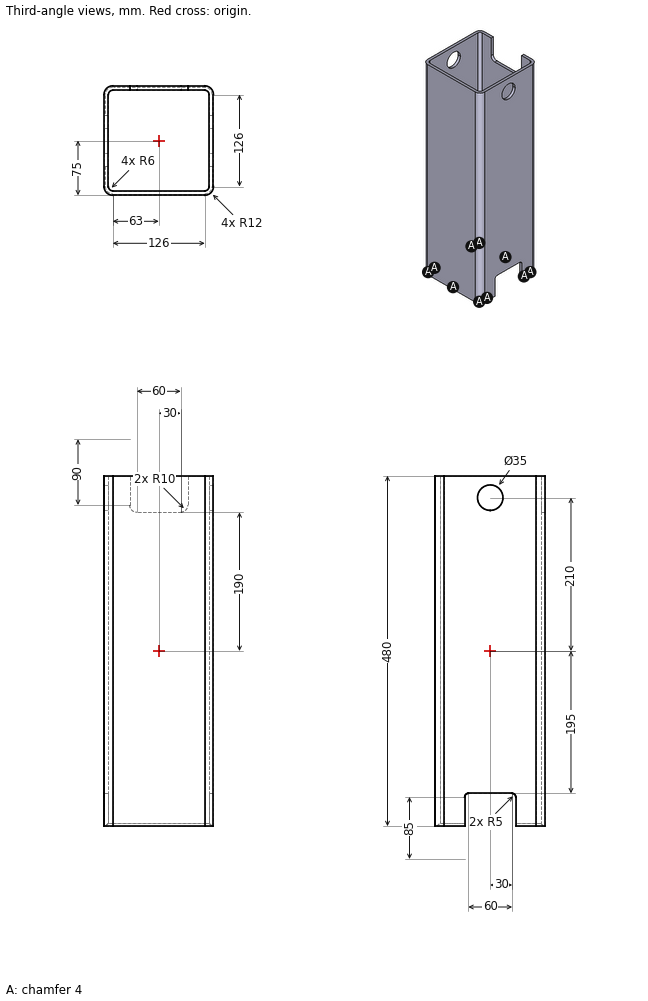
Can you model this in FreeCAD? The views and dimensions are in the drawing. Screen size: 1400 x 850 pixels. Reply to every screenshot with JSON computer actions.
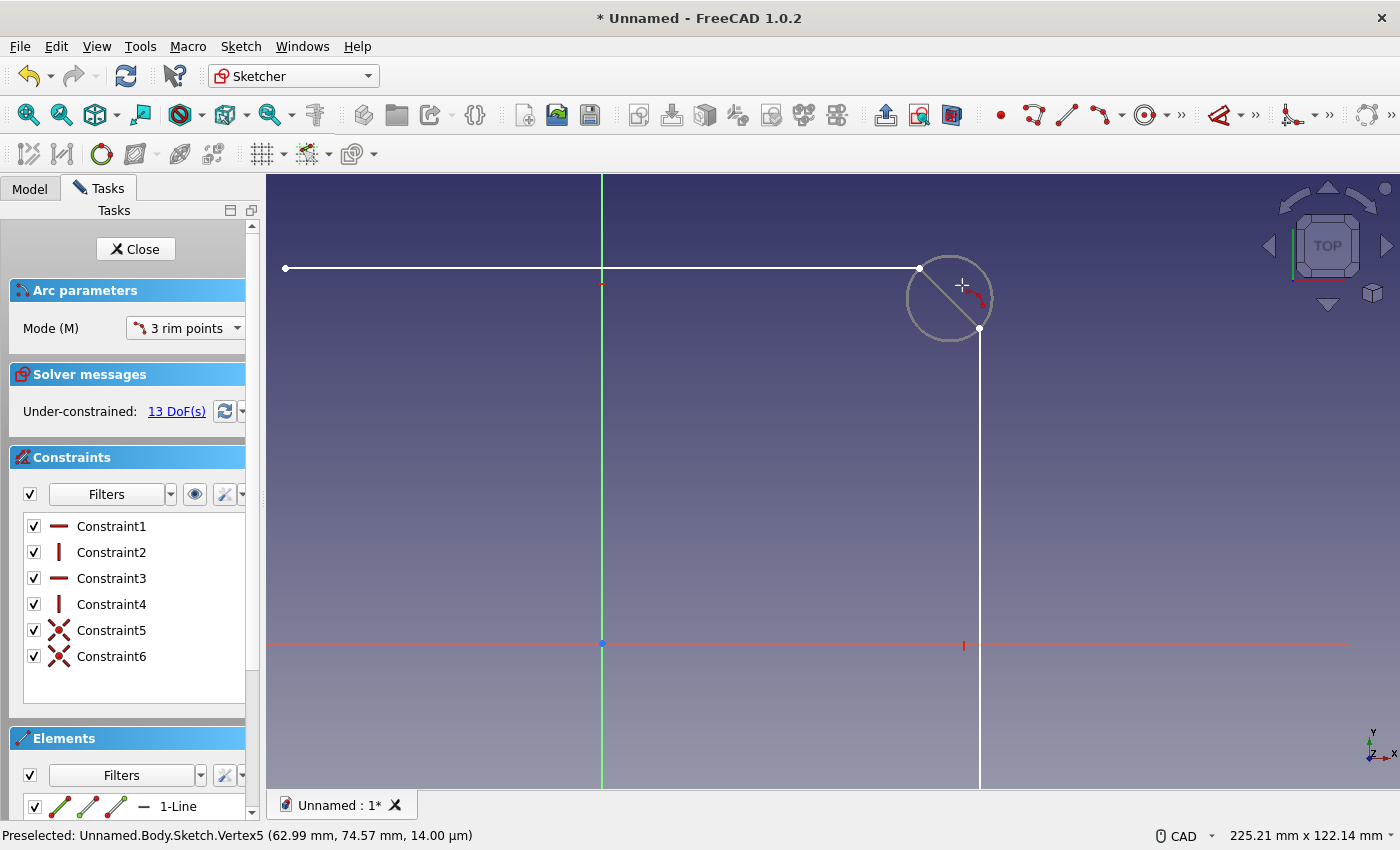
{"action": "left_click", "coordinate": [962, 284]}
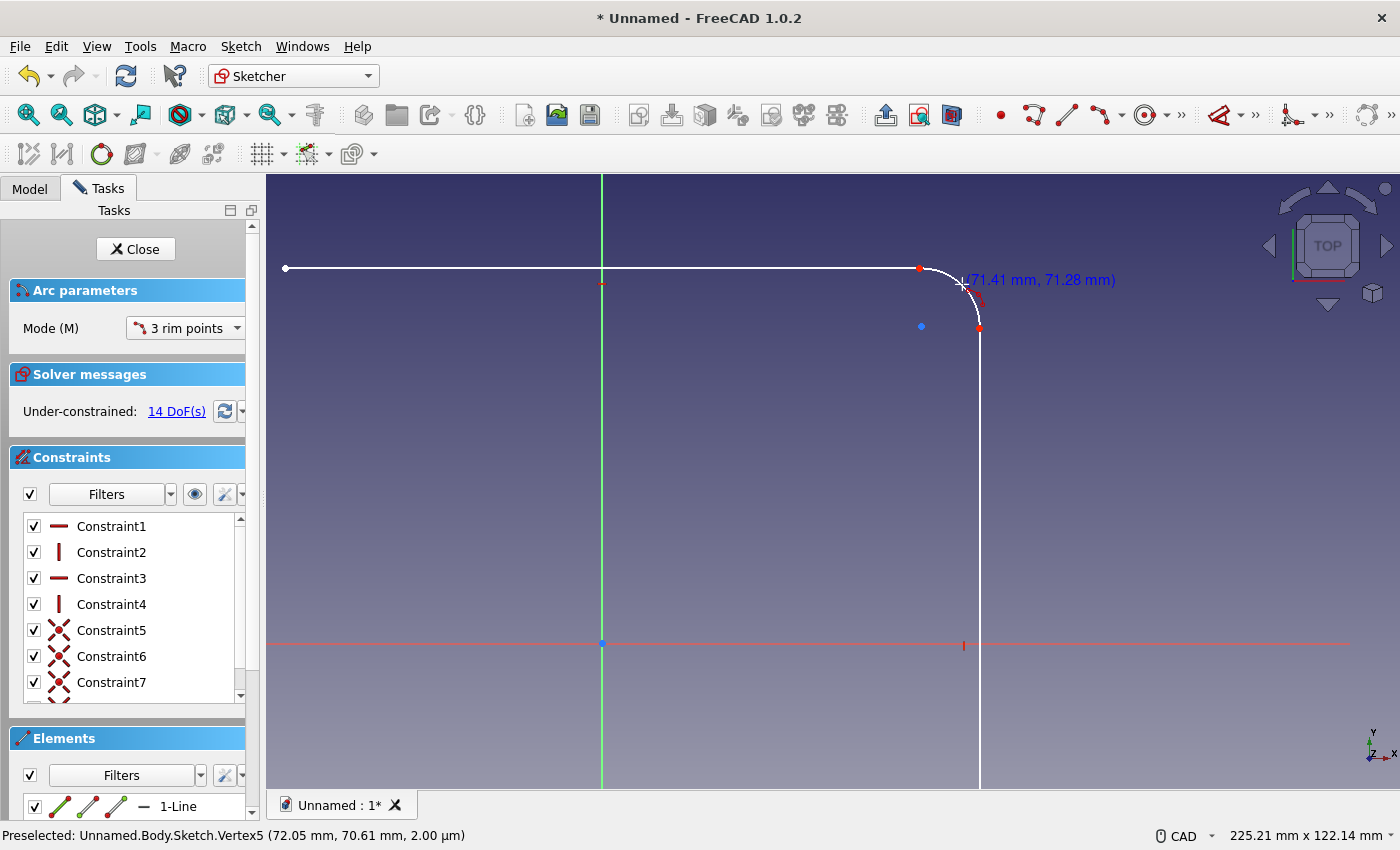
{"action": "scroll", "coordinate": [962, 284], "scroll_direction": "down", "scroll_amount": 3}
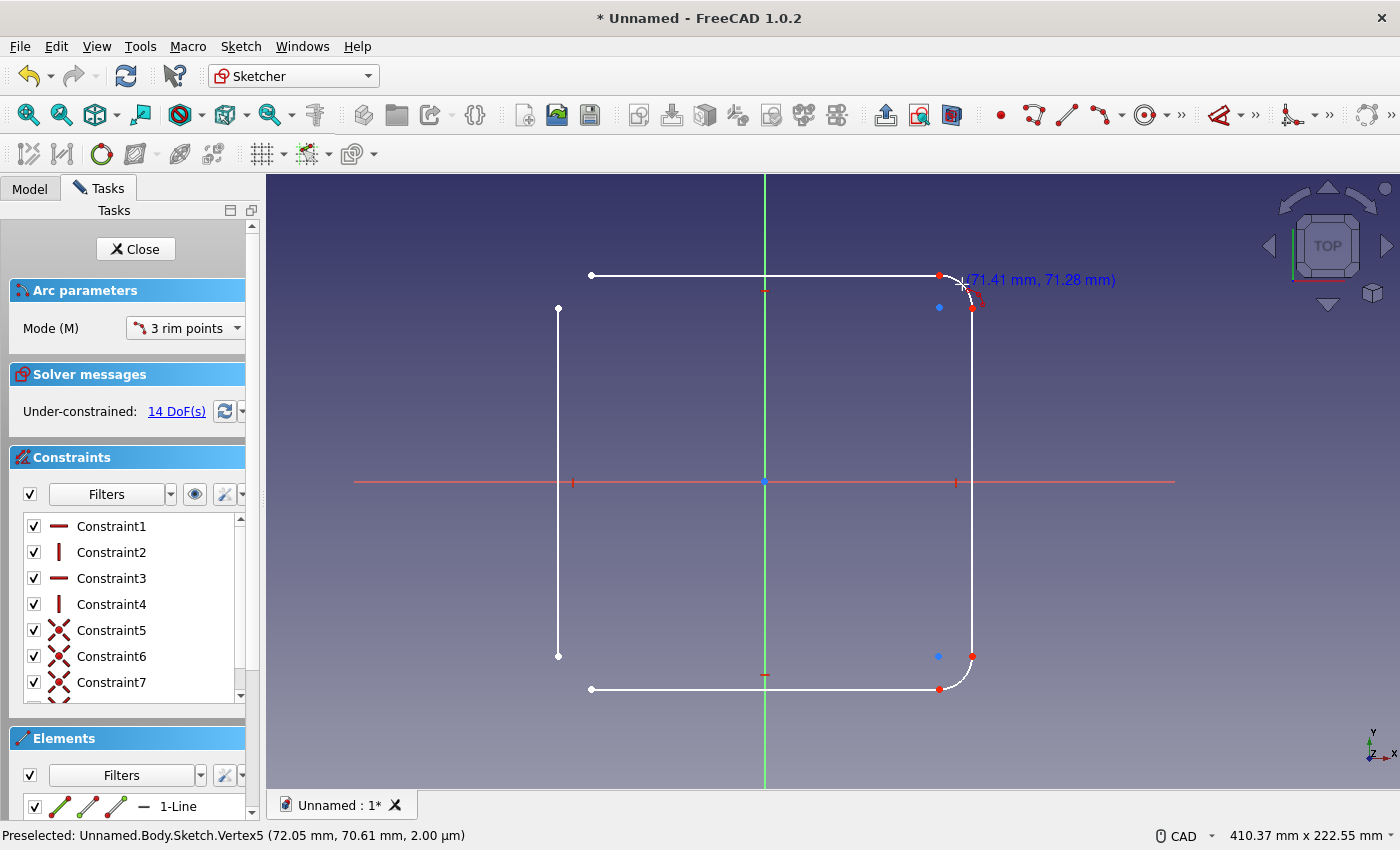
{"action": "left_click", "coordinate": [591, 276]}
{"action": "left_click", "coordinate": [558, 309]}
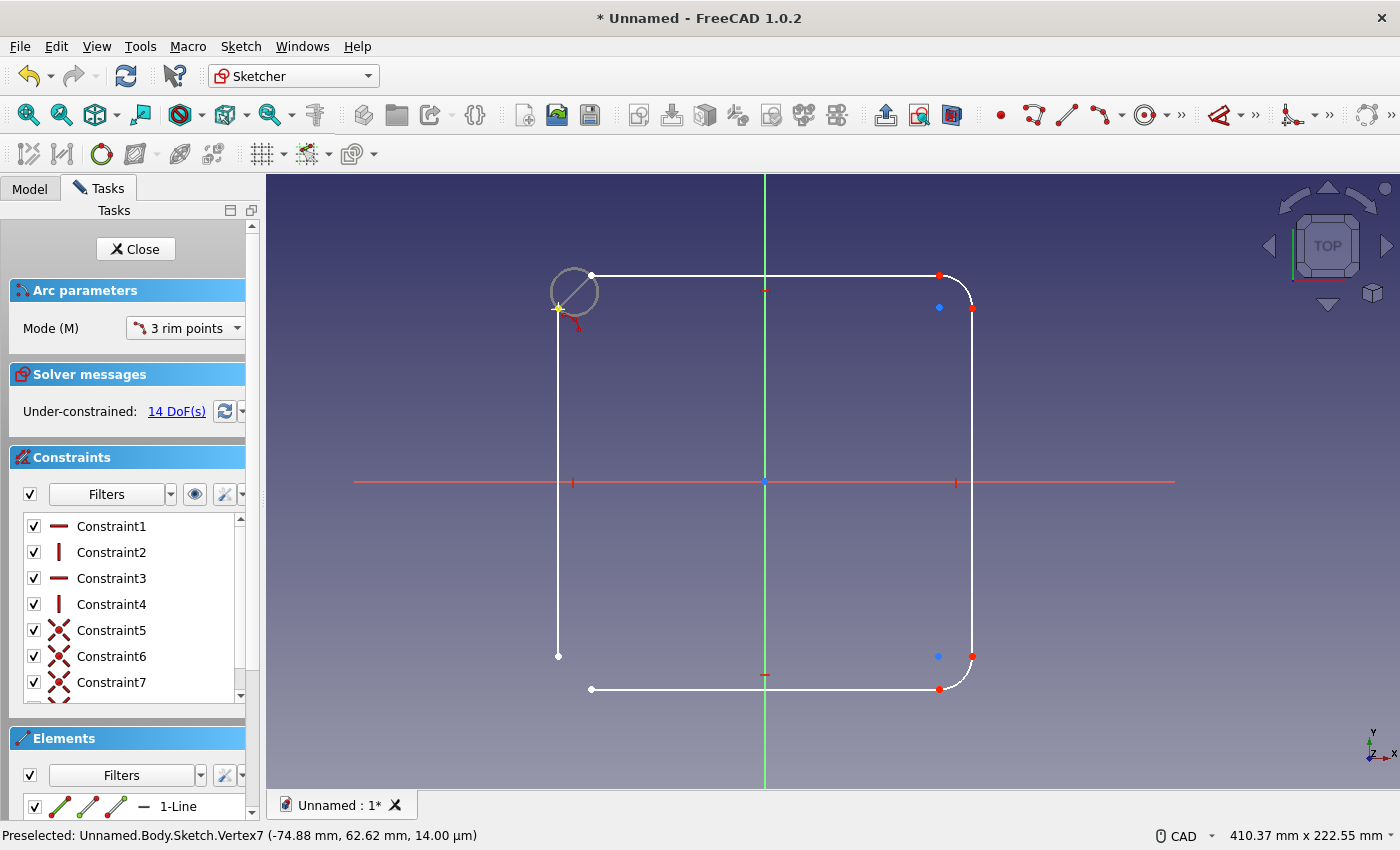
{"action": "scroll", "coordinate": [567, 284], "scroll_direction": "up", "scroll_amount": 3}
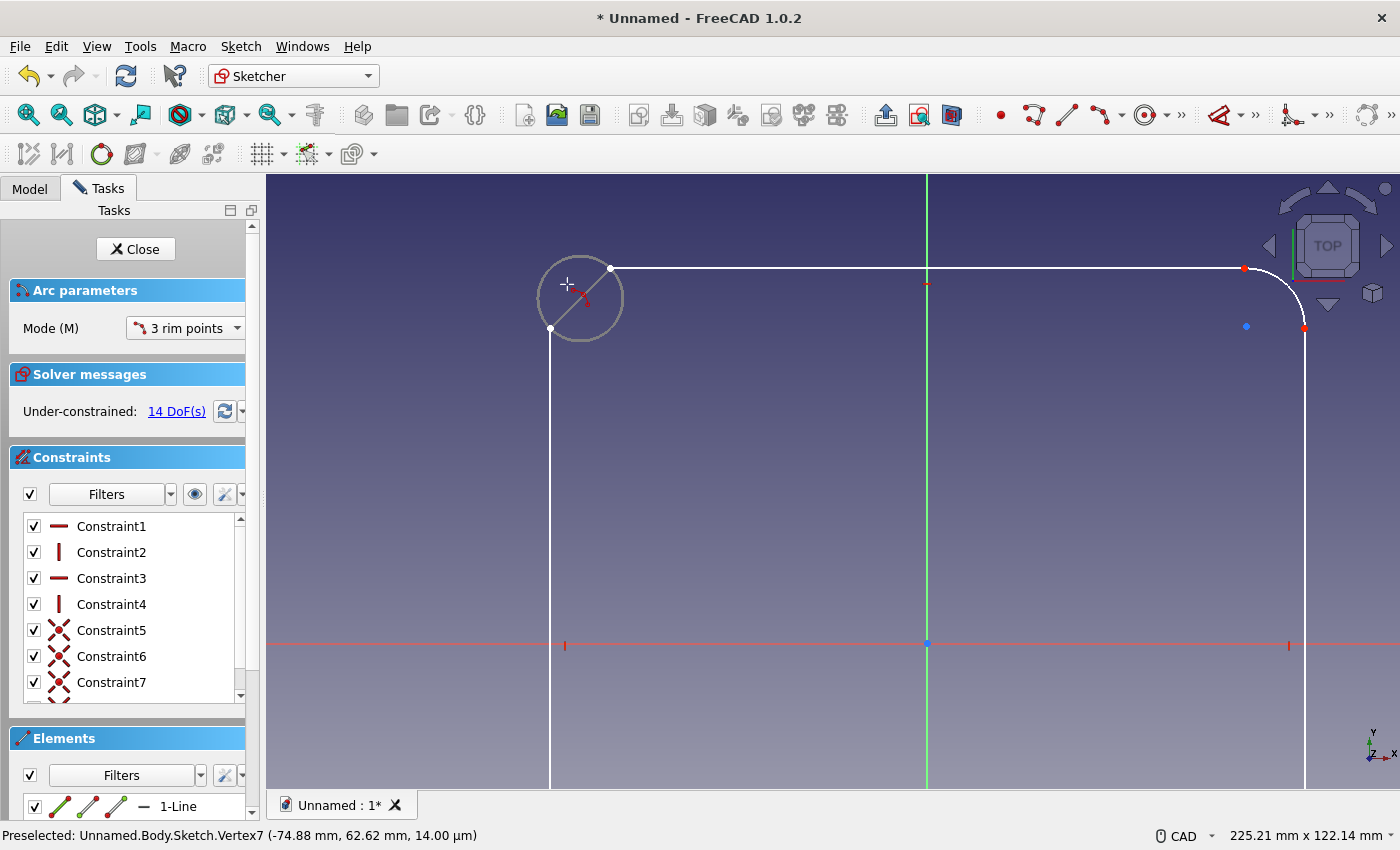
{"action": "left_click", "coordinate": [567, 284]}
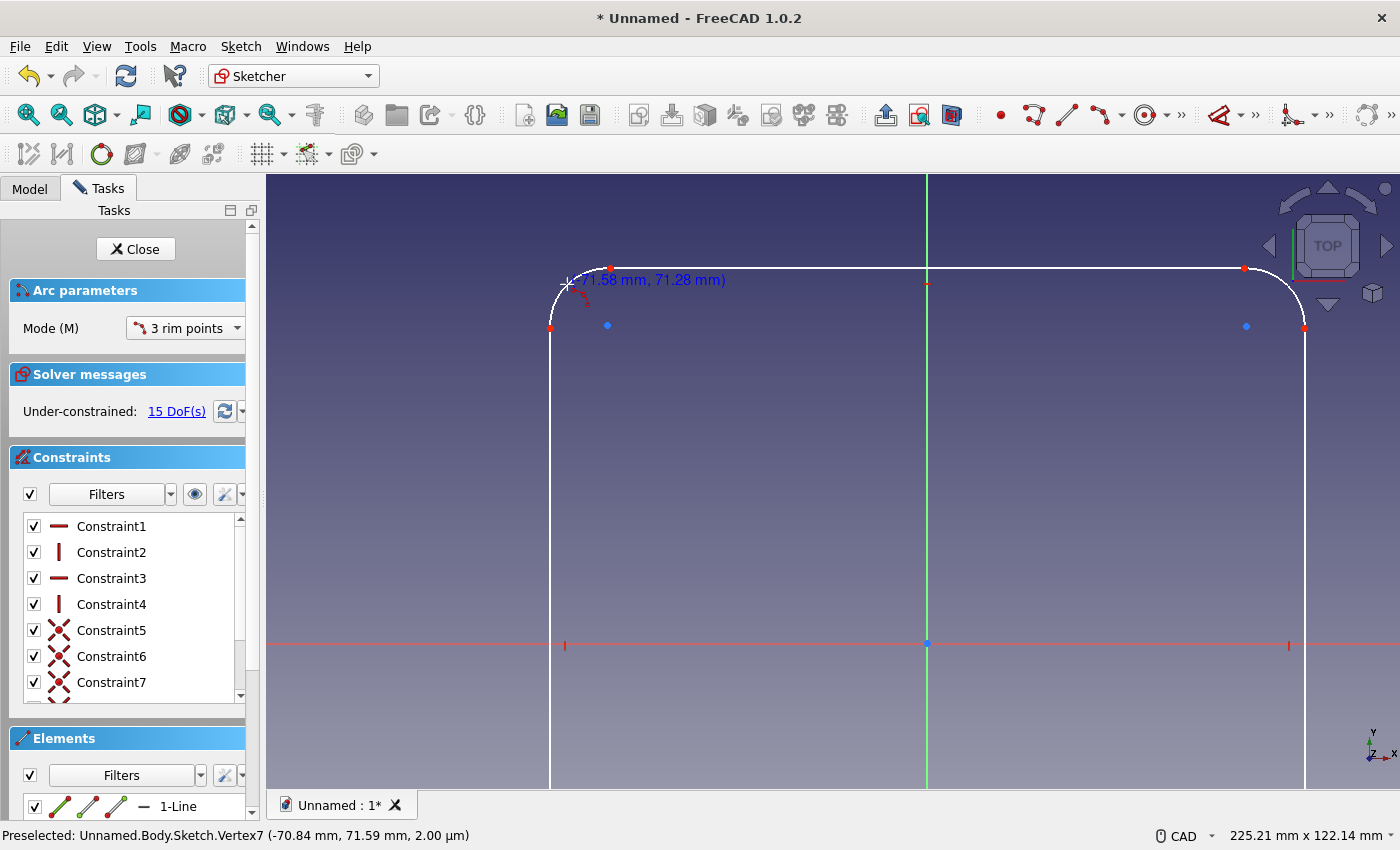
{"action": "scroll", "coordinate": [566, 284], "scroll_direction": "down", "scroll_amount": 3}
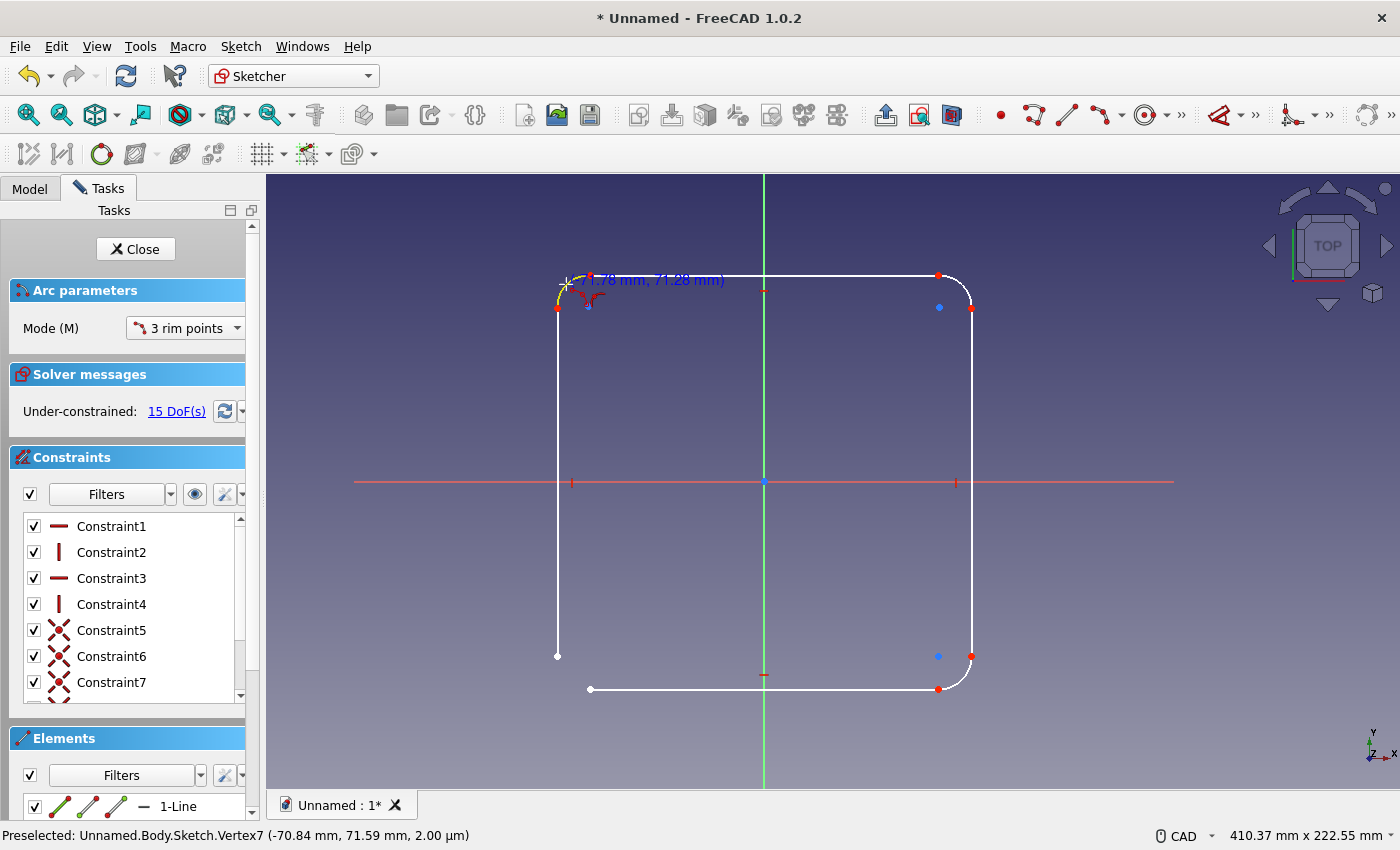
{"action": "left_click", "coordinate": [558, 657]}
{"action": "left_click", "coordinate": [591, 690]}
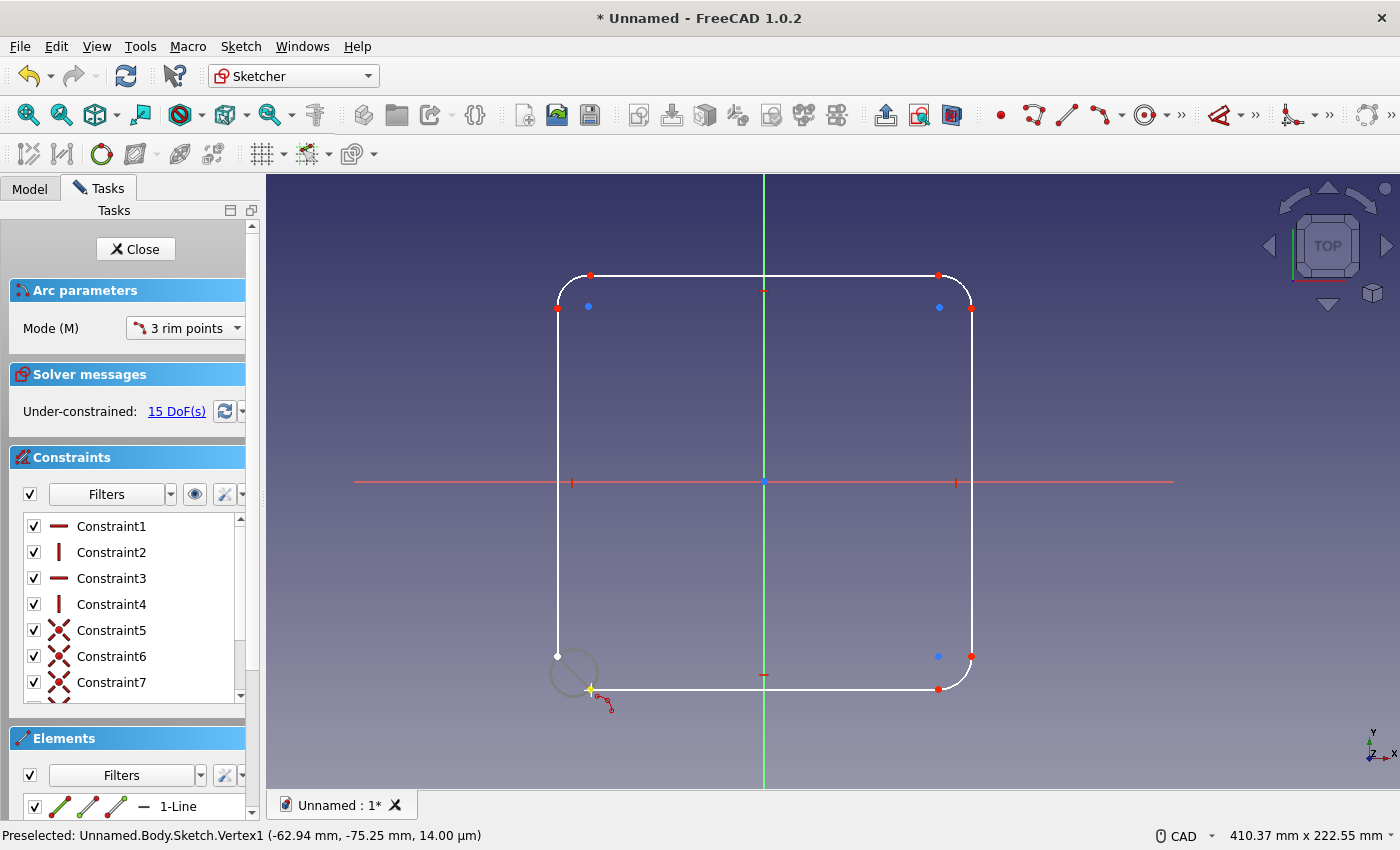
{"action": "scroll", "coordinate": [567, 679], "scroll_direction": "up", "scroll_amount": 3}